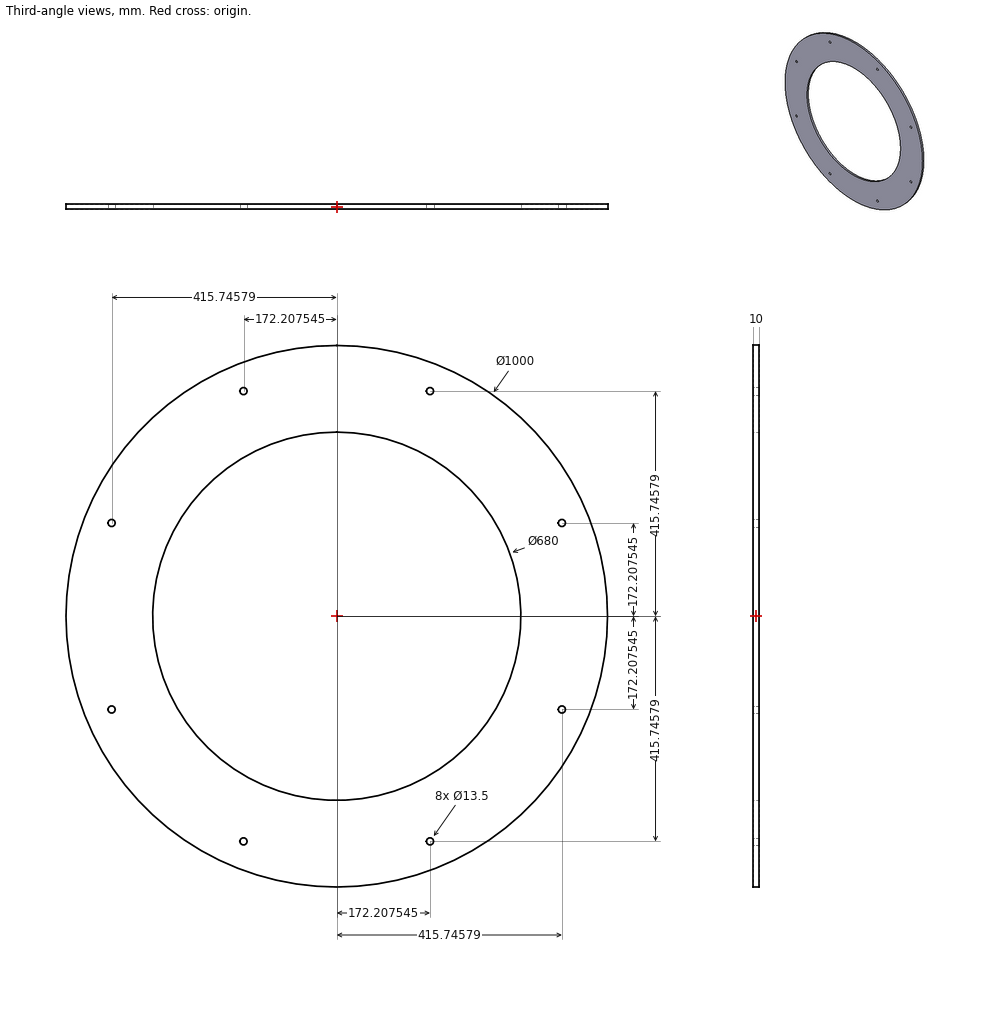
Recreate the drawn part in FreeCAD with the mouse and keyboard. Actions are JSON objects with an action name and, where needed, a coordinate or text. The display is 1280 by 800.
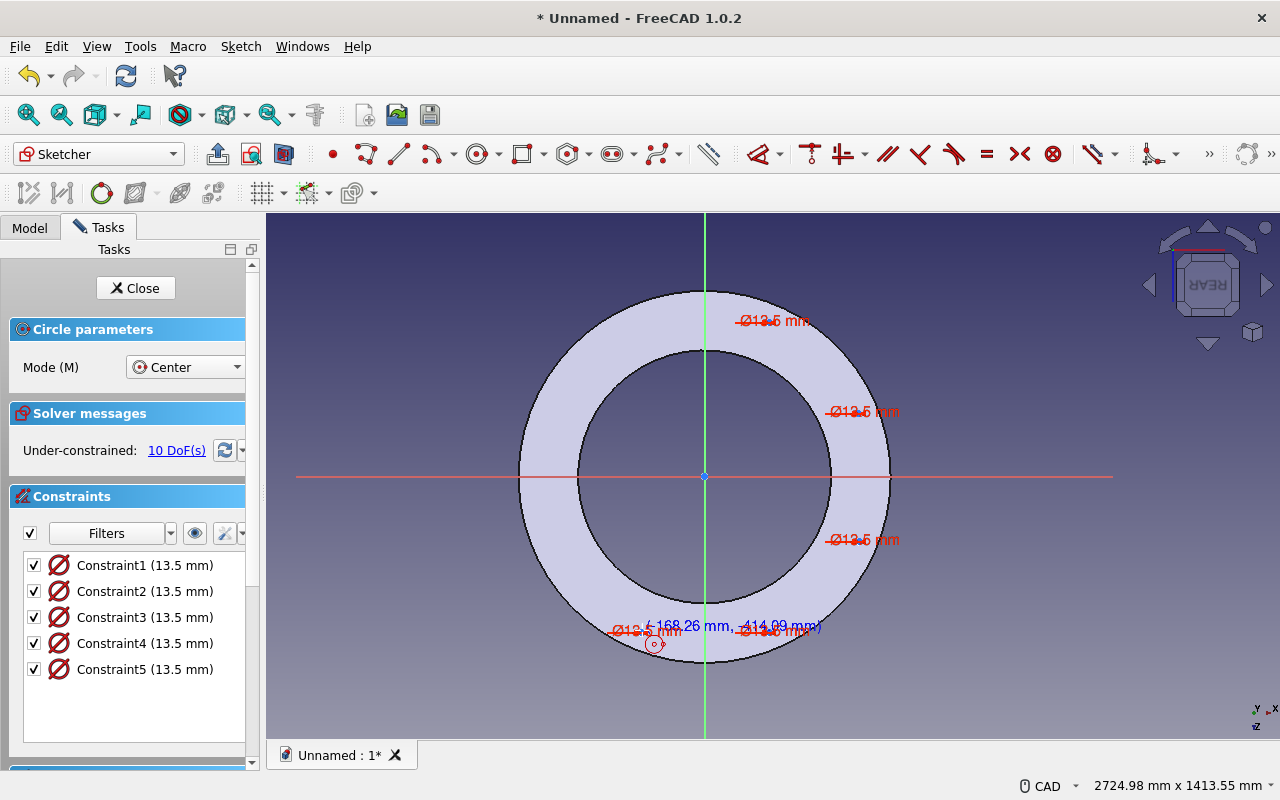
{"action": "scroll", "coordinate": [550, 541], "scroll_direction": "up", "scroll_amount": 12}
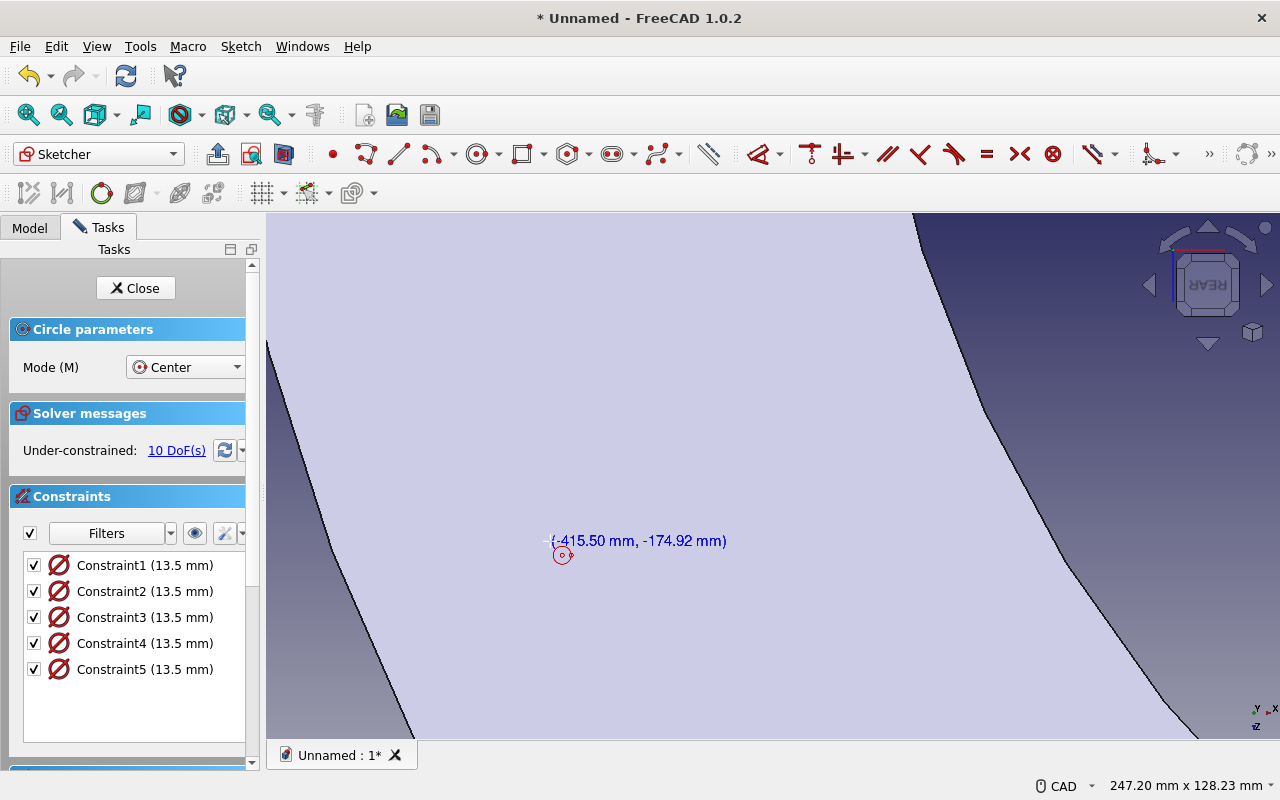
{"action": "scroll", "coordinate": [550, 541], "scroll_direction": "down", "scroll_amount": 12}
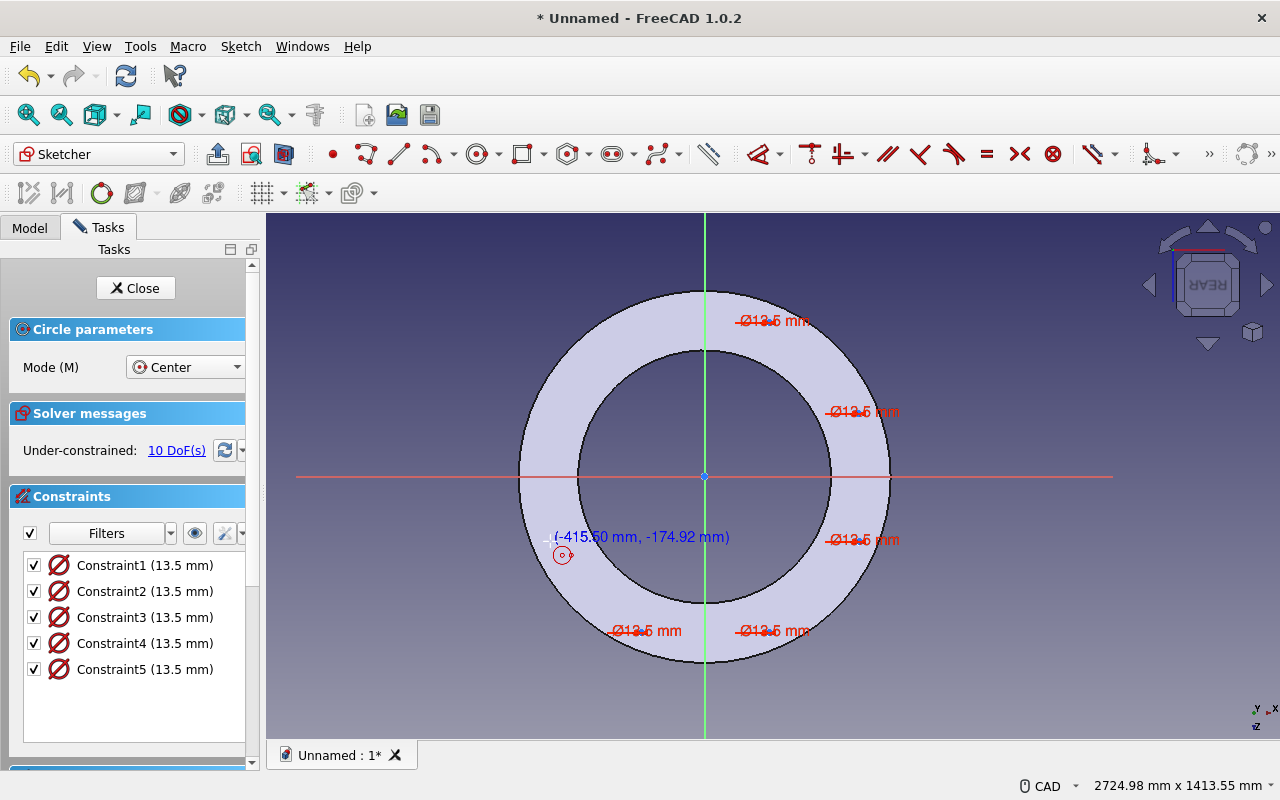
{"action": "left_click", "coordinate": [550, 541]}
{"action": "mouse_move", "coordinate": [552, 539]}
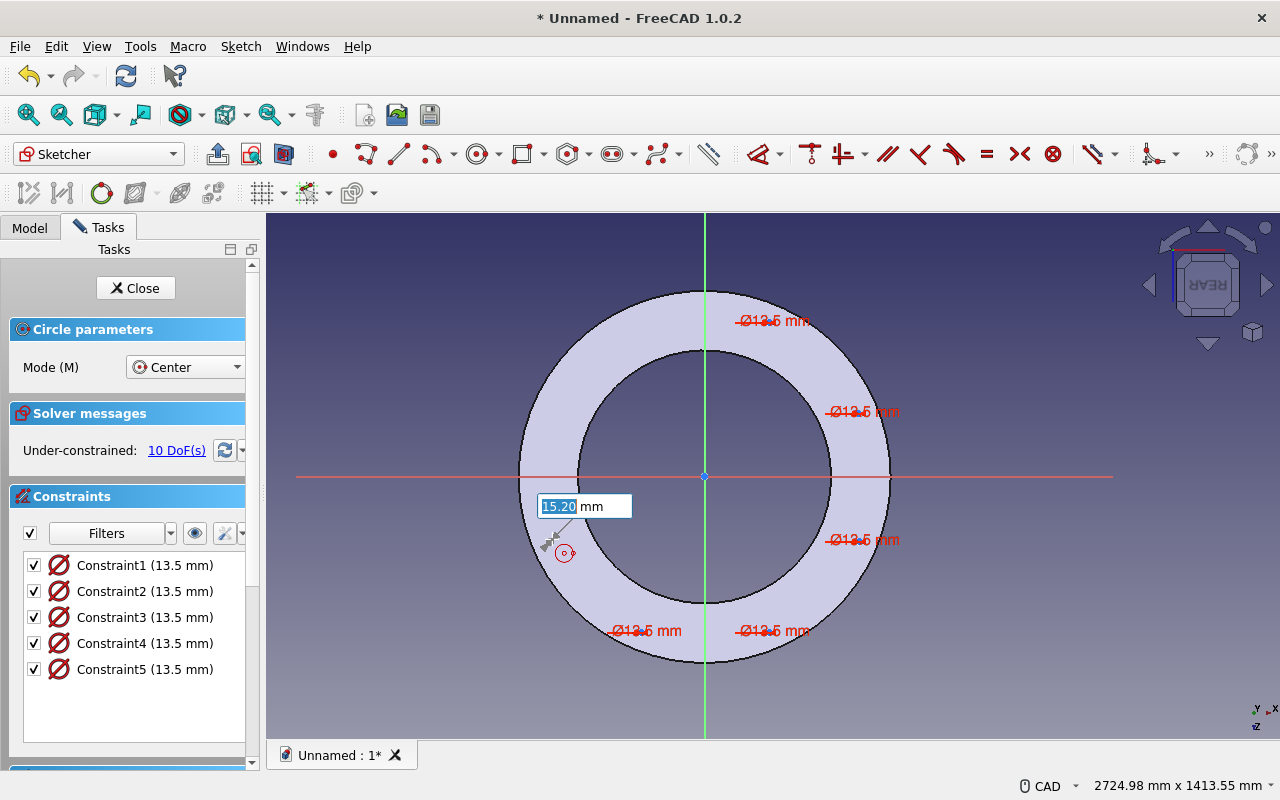
{"action": "type", "text": "13.5"}
{"action": "key", "text": "Return"}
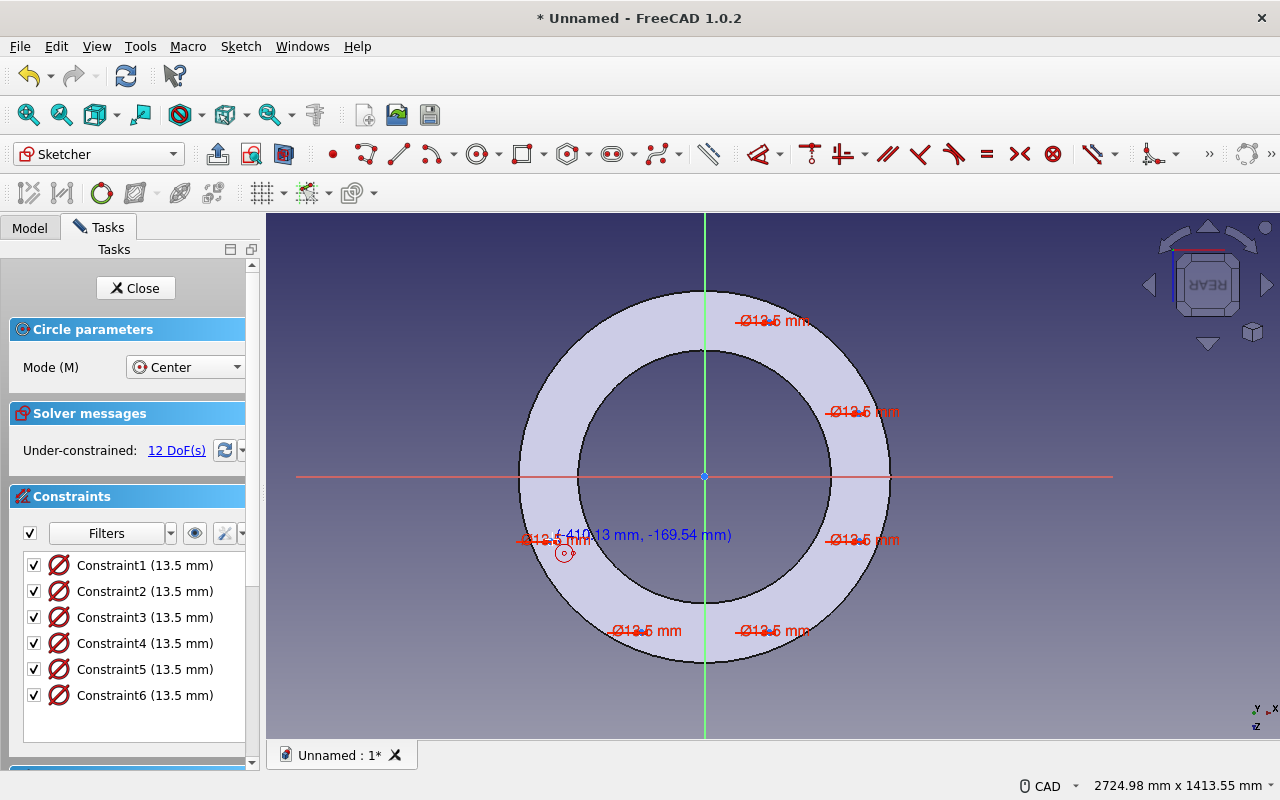
{"action": "scroll", "coordinate": [550, 413], "scroll_direction": "up", "scroll_amount": 12}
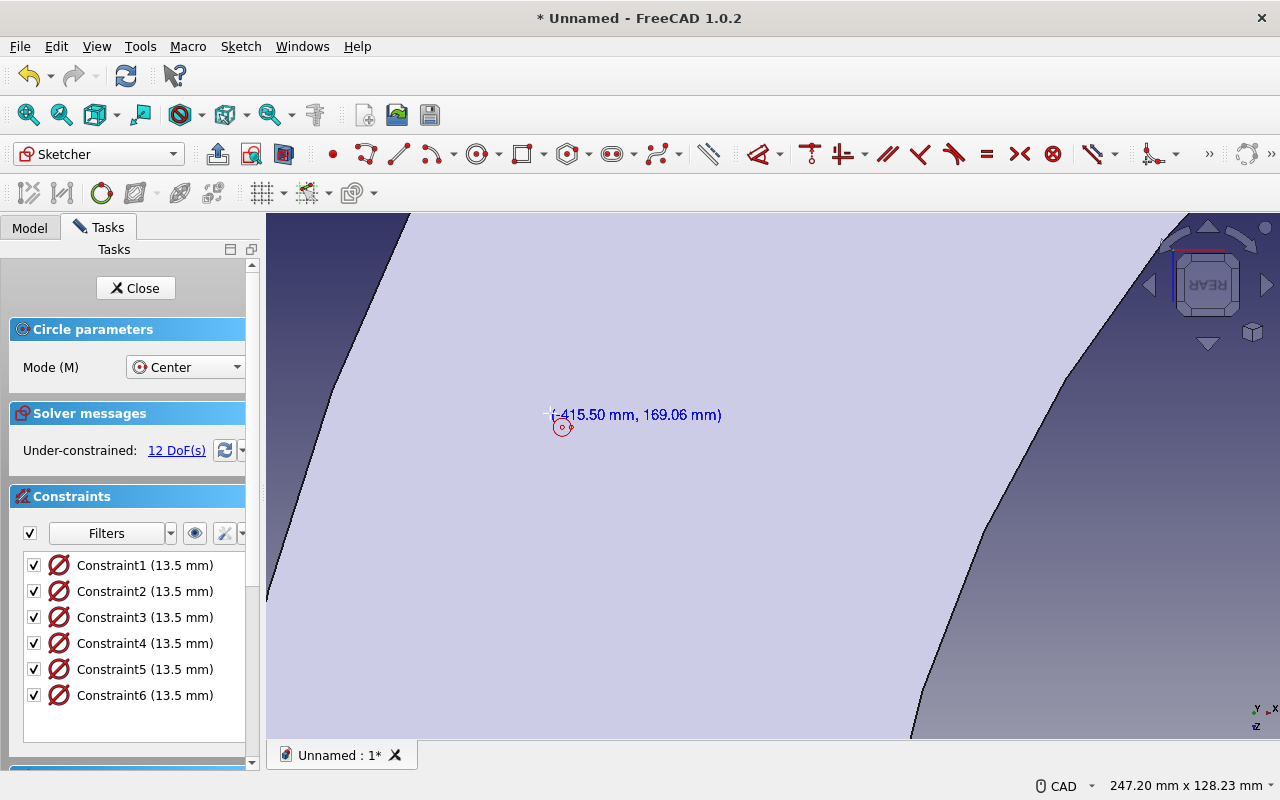
{"action": "scroll", "coordinate": [550, 412], "scroll_direction": "down", "scroll_amount": 12}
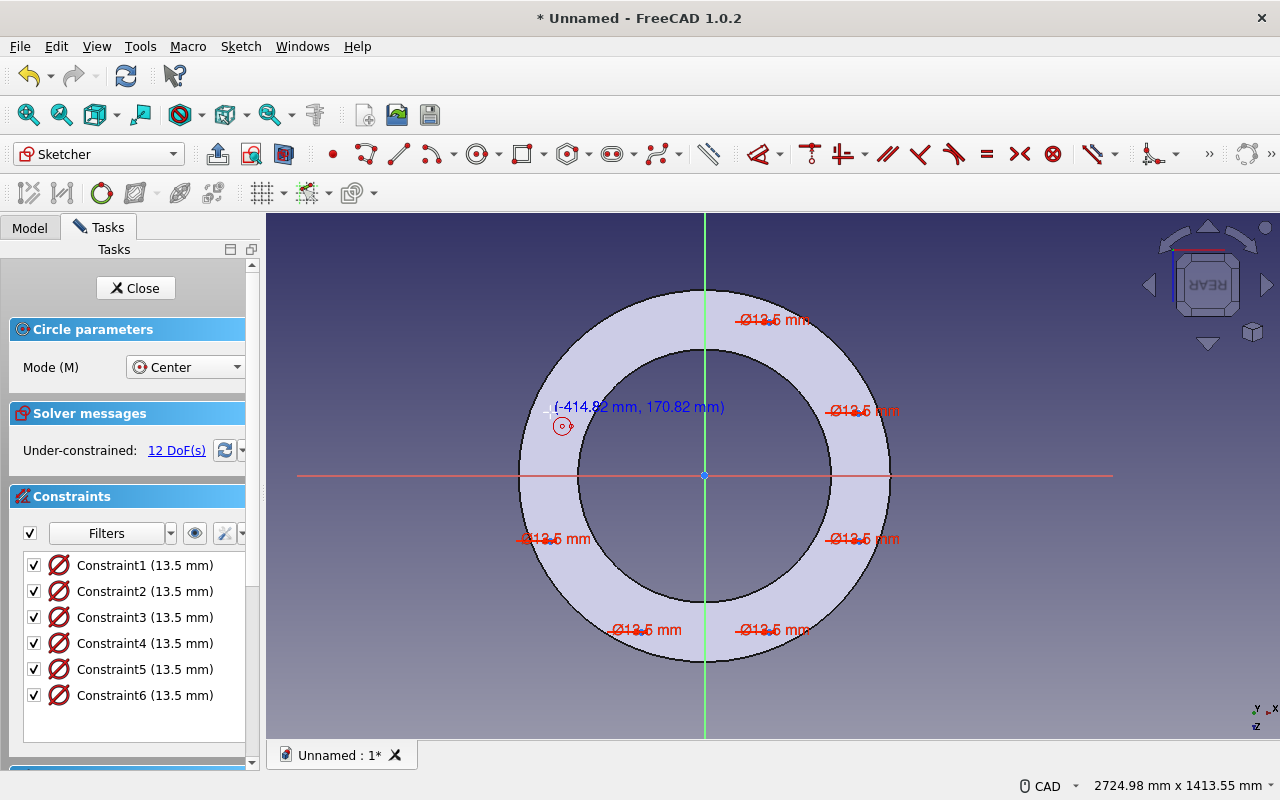
{"action": "left_click", "coordinate": [550, 412]}
{"action": "mouse_move", "coordinate": [552, 410]}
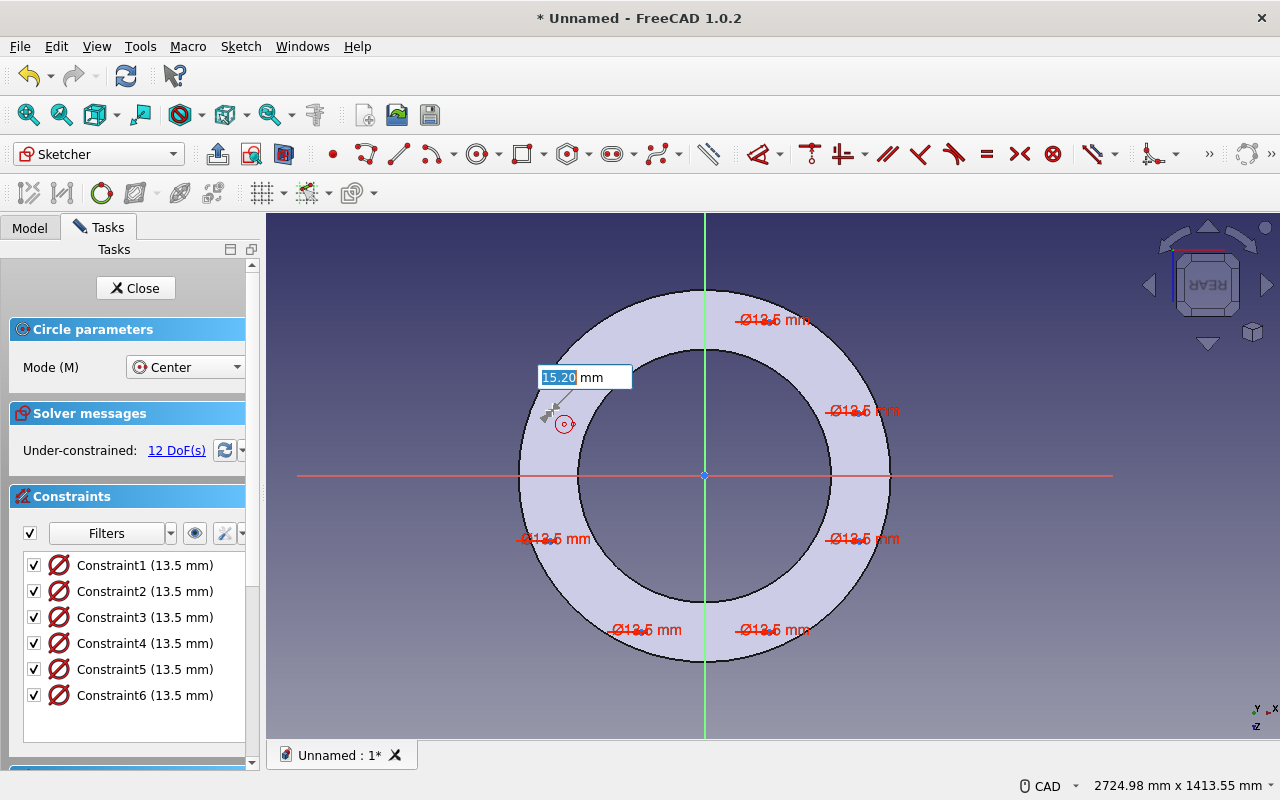
{"action": "type", "text": "13.5"}
{"action": "key", "text": "Return"}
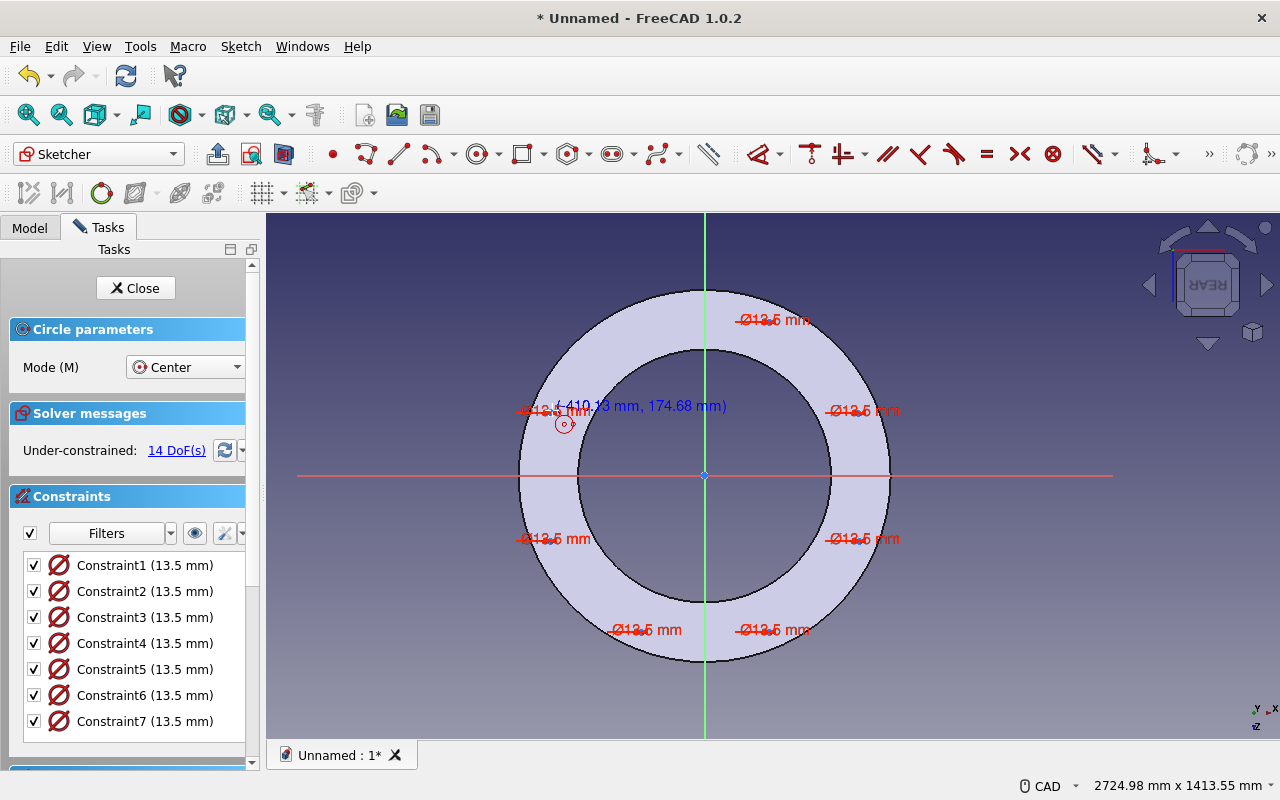
{"action": "scroll", "coordinate": [641, 321], "scroll_direction": "up", "scroll_amount": 12}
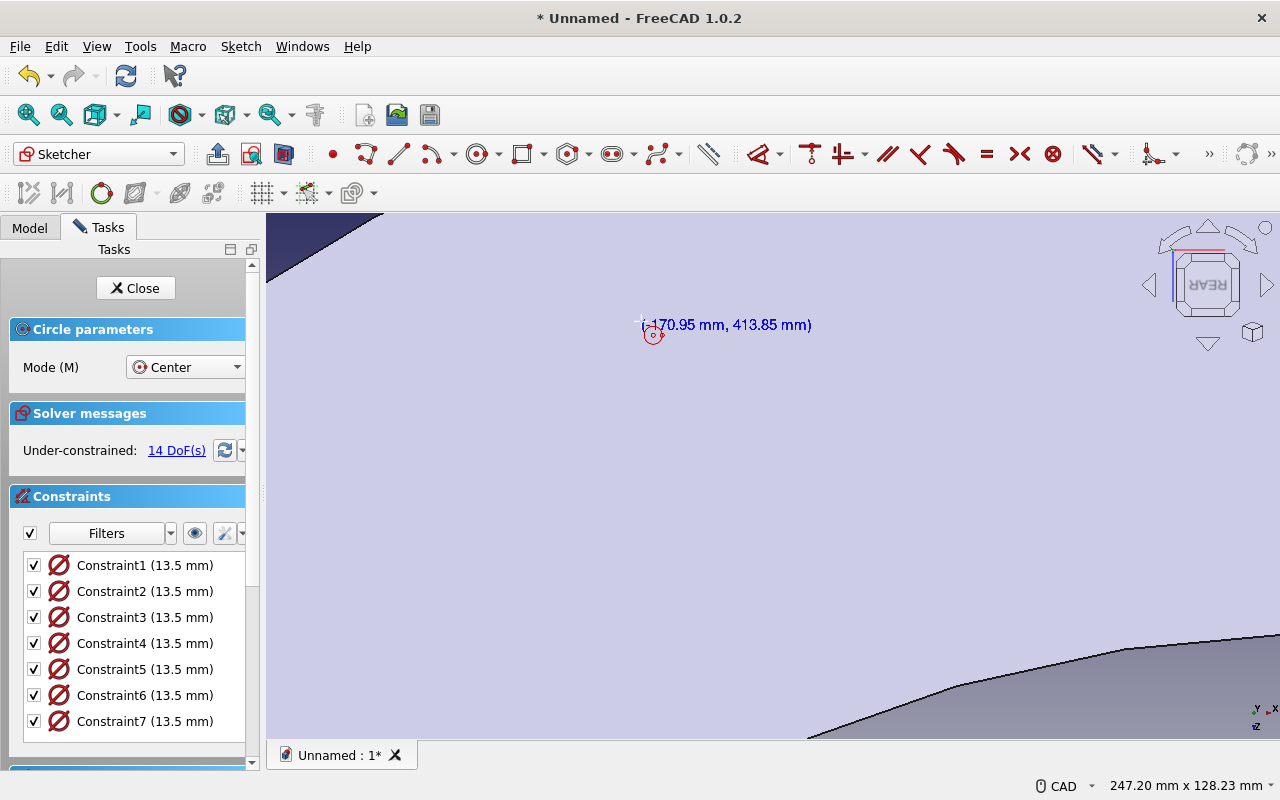
{"action": "scroll", "coordinate": [641, 321], "scroll_direction": "down", "scroll_amount": 12}